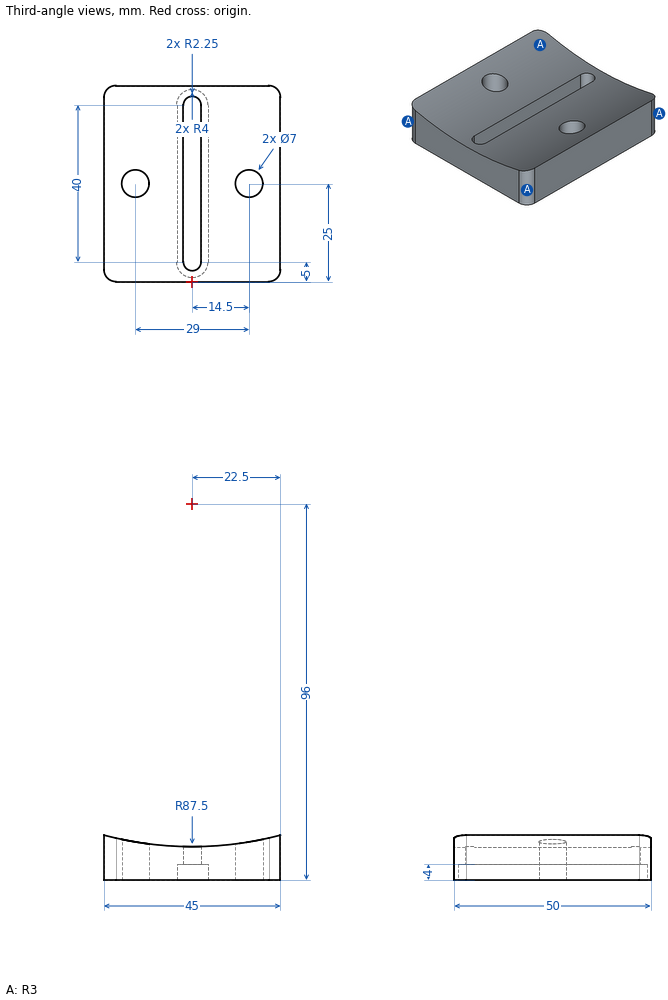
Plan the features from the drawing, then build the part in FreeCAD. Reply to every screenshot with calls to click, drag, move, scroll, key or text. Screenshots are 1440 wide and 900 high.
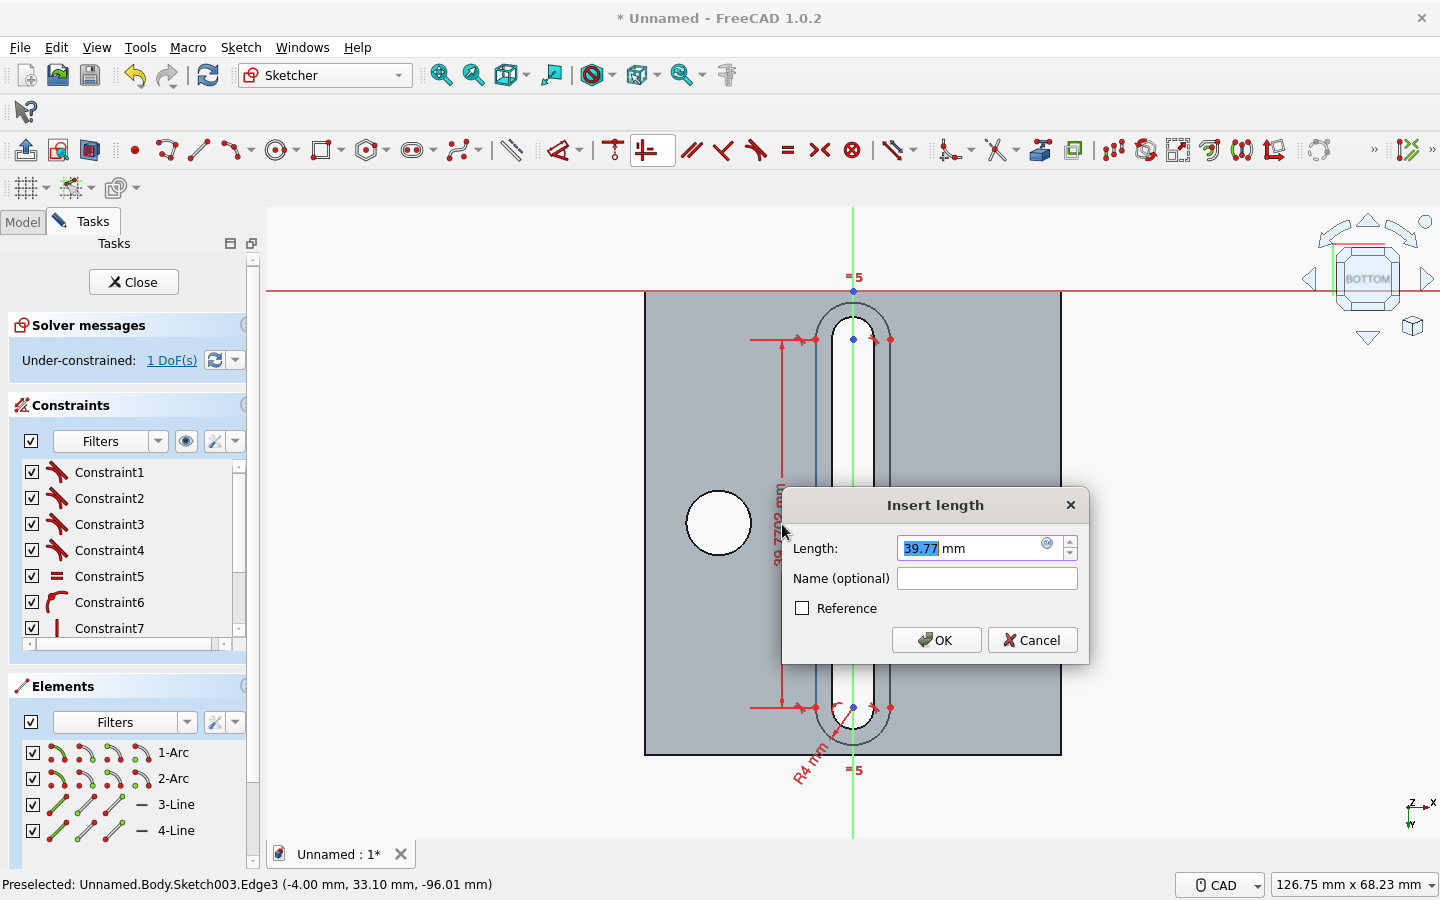
text(40)
key(Return)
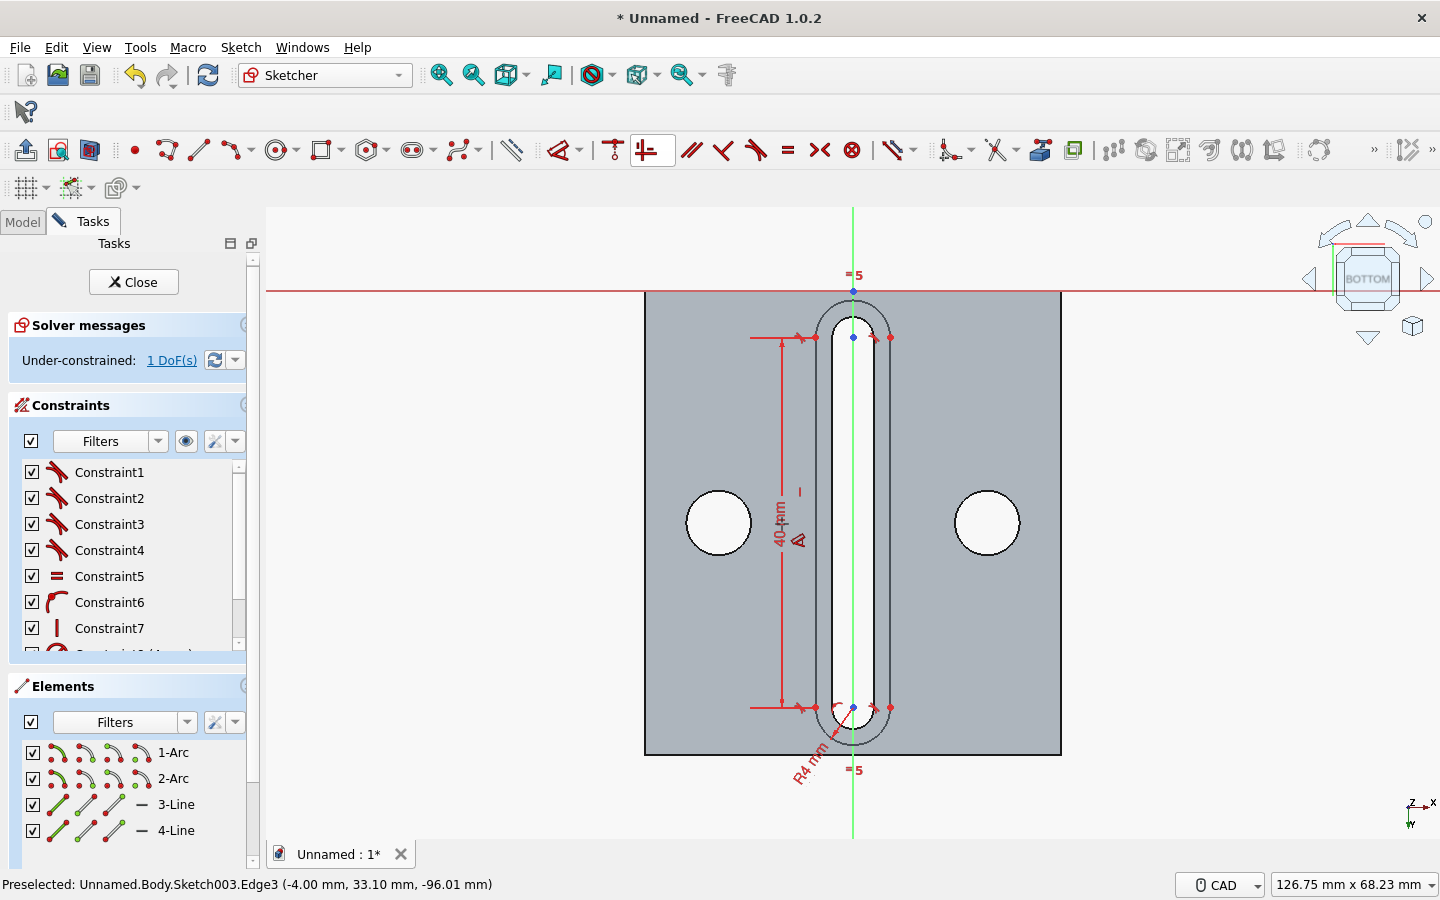
click(890, 338)
click(924, 314)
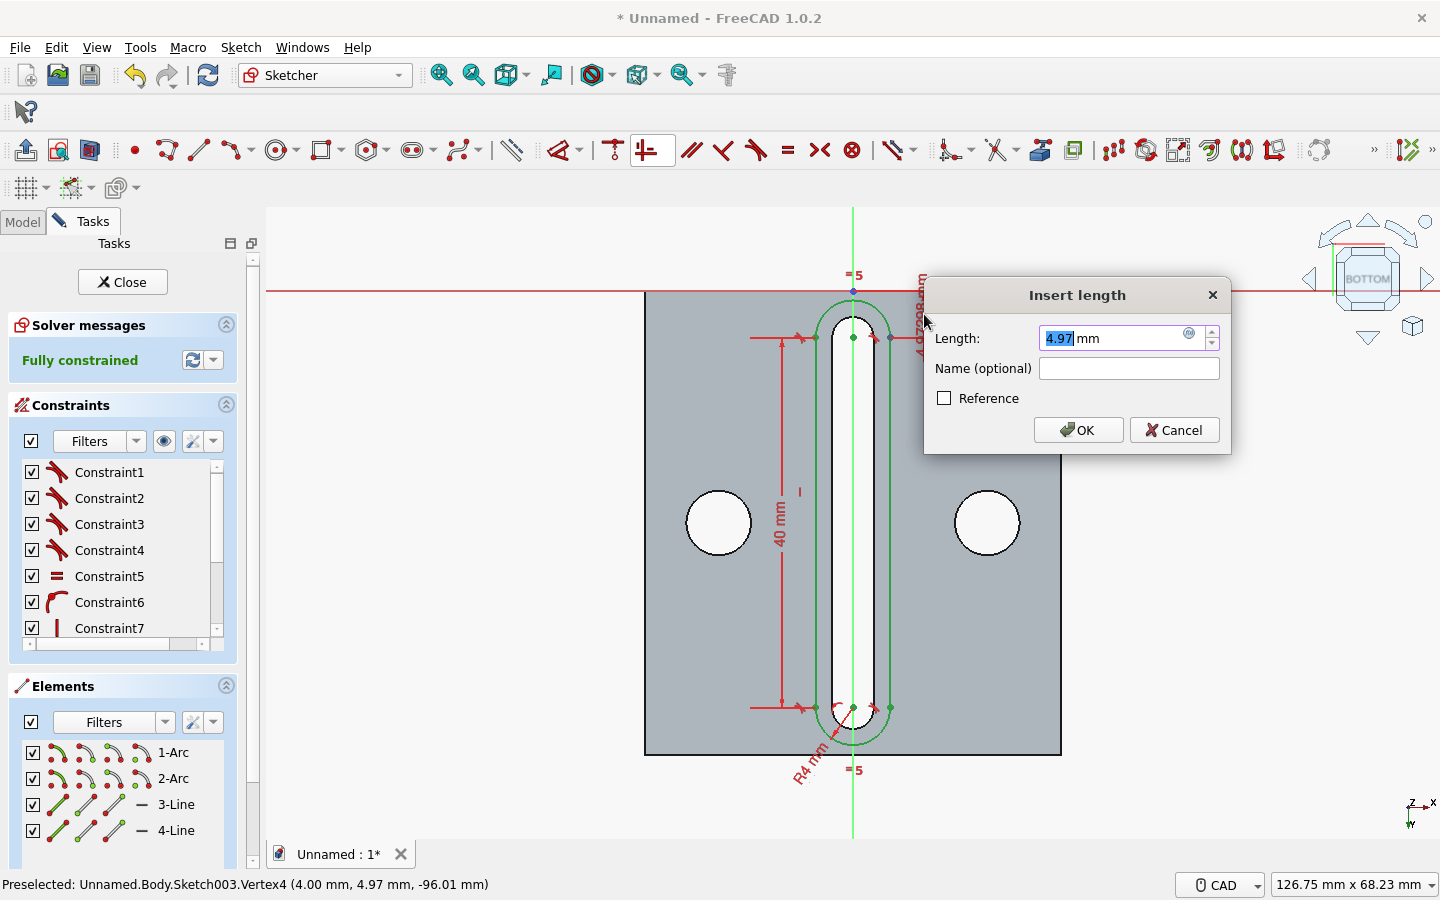
text(5)
key(Return)
key(Escape)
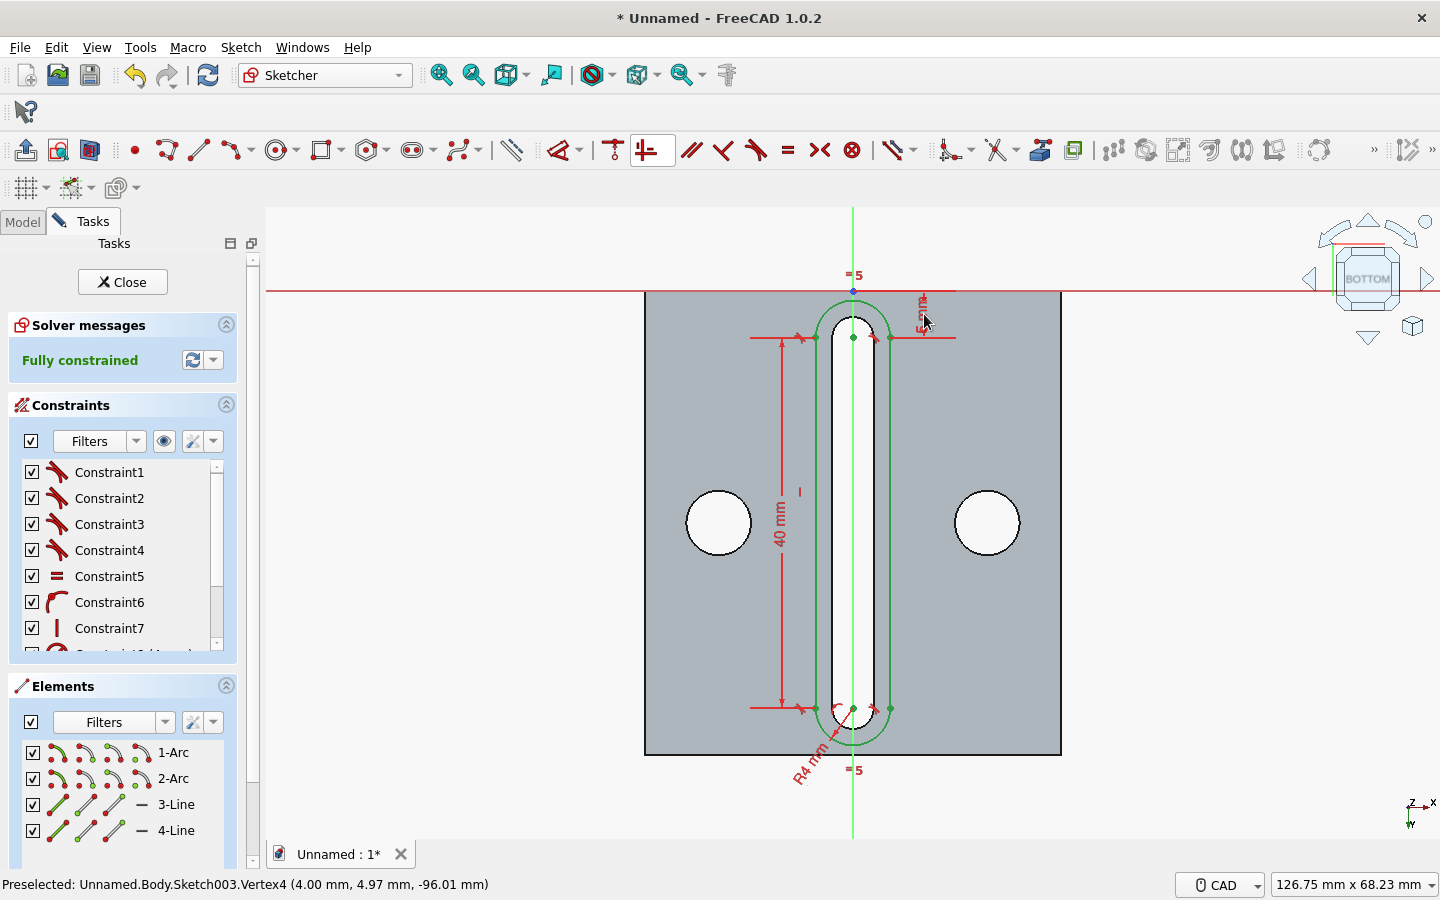
click(123, 282)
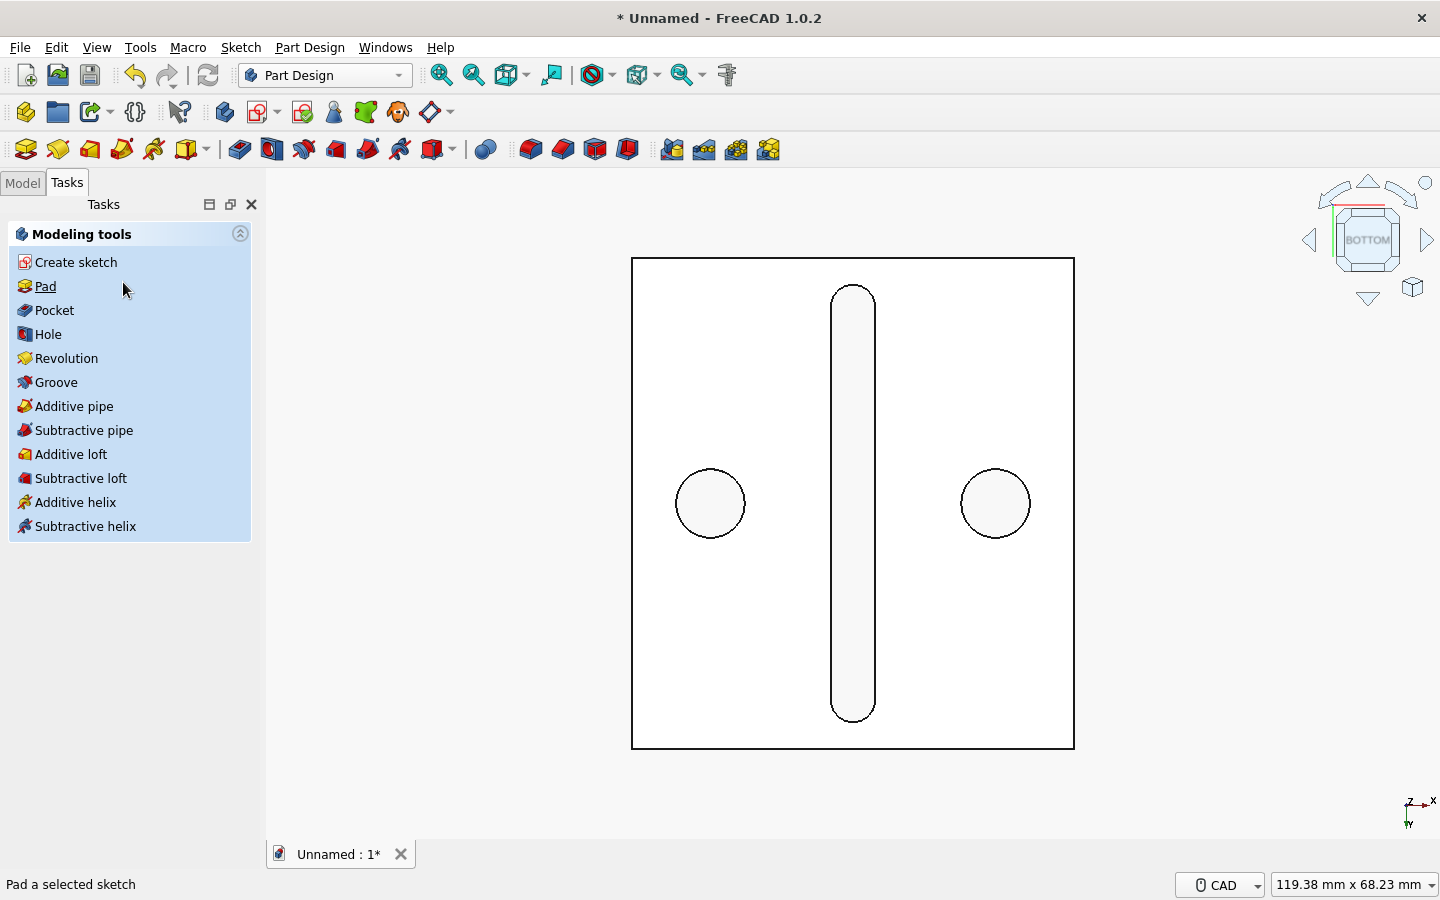
click(240, 150)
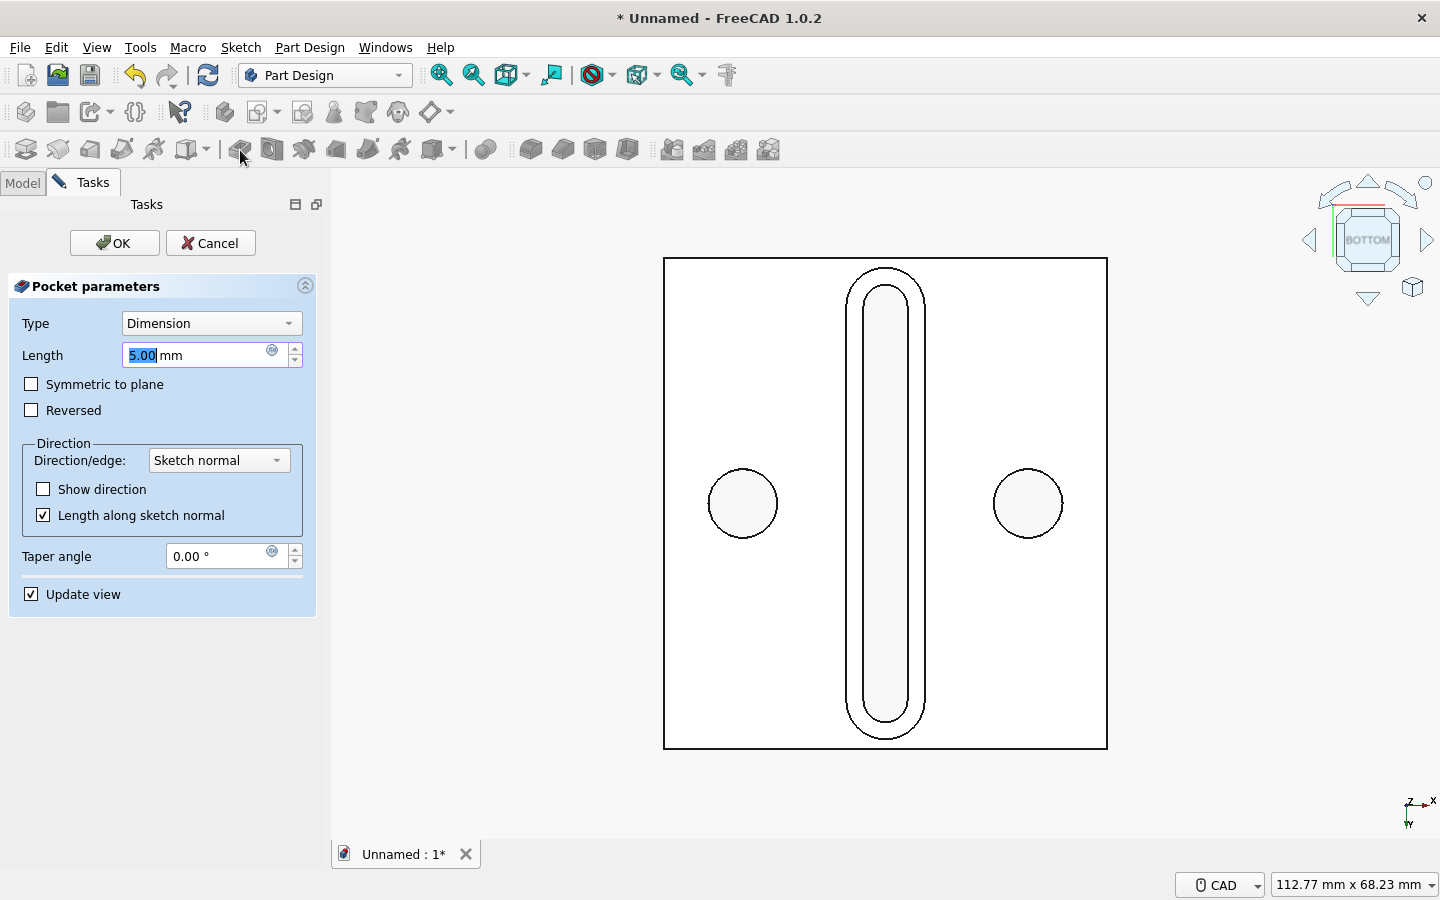
text(4)
key(Tab)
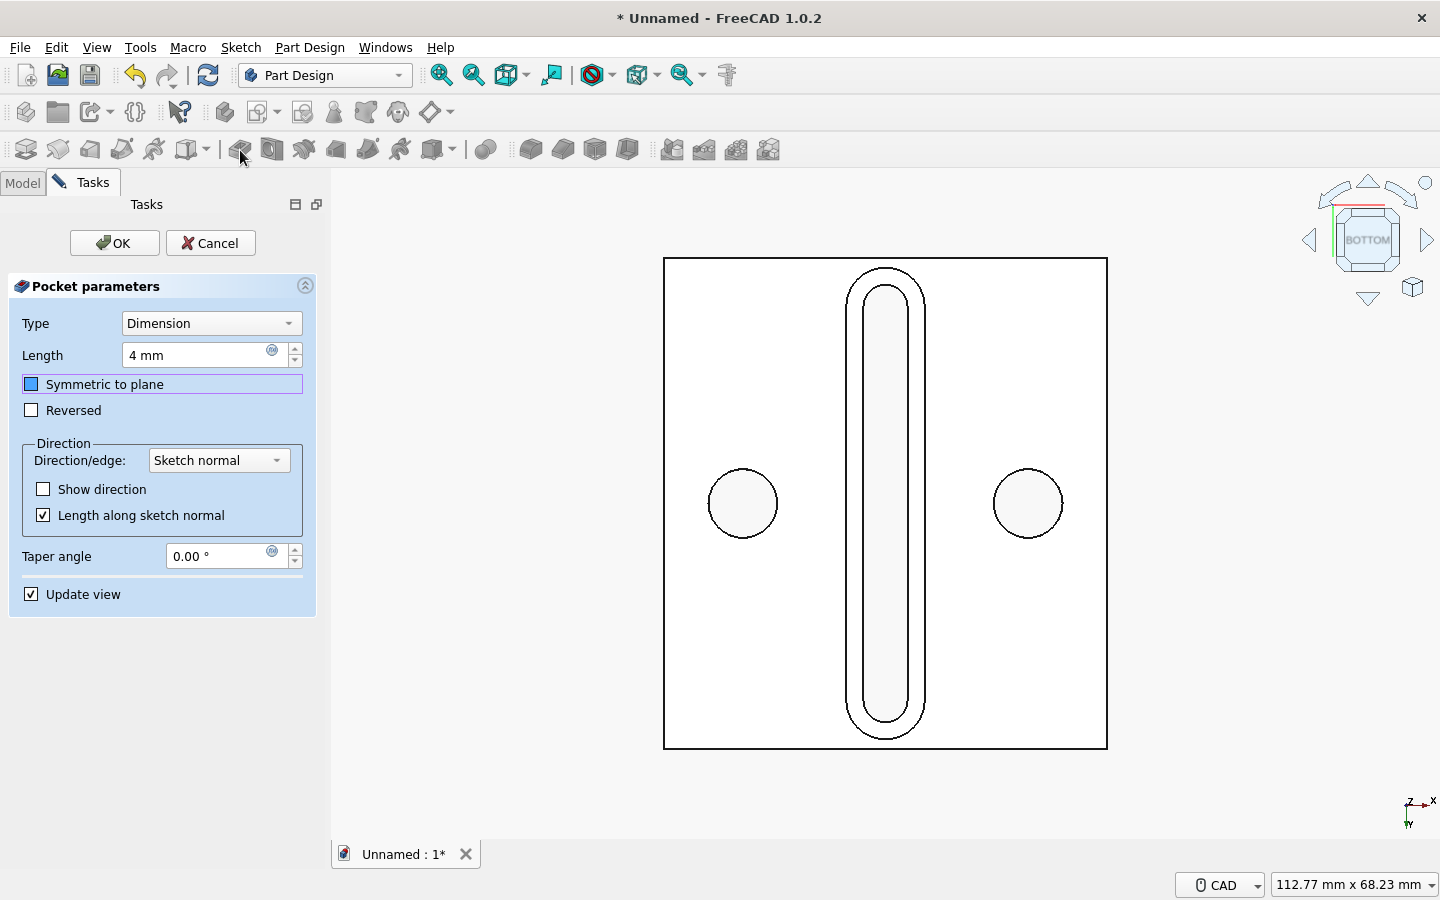
click(115, 243)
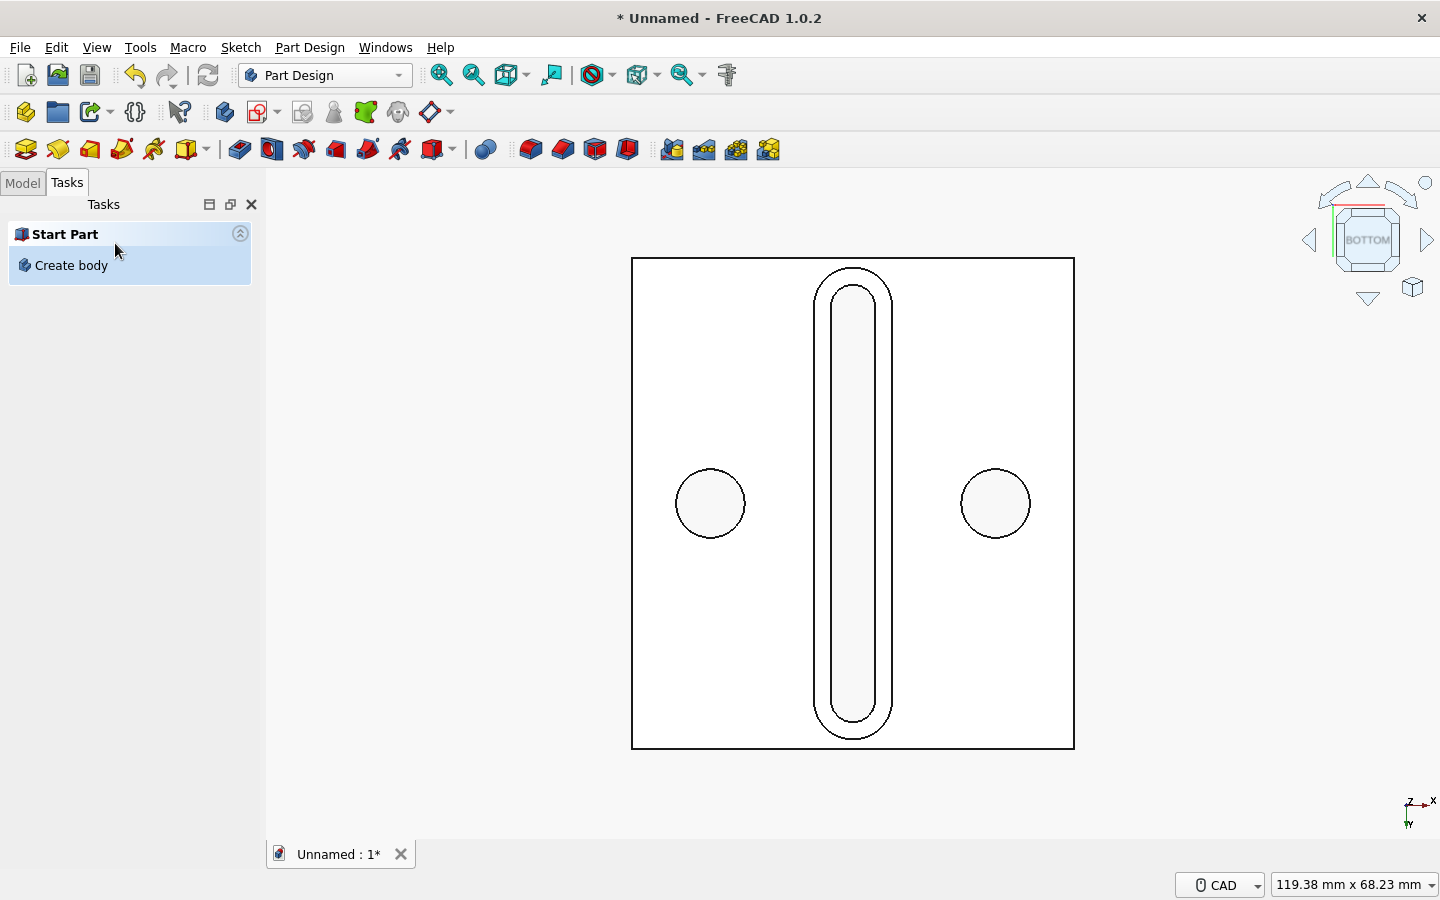
key(0)